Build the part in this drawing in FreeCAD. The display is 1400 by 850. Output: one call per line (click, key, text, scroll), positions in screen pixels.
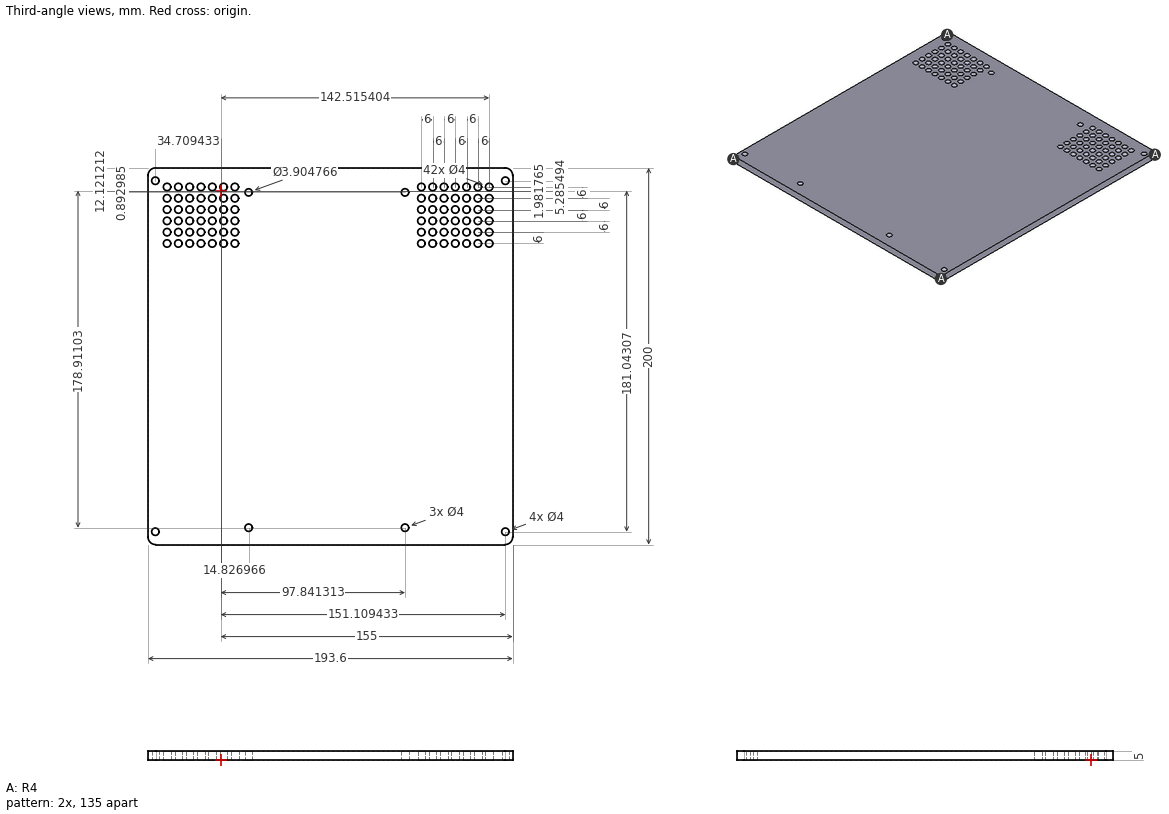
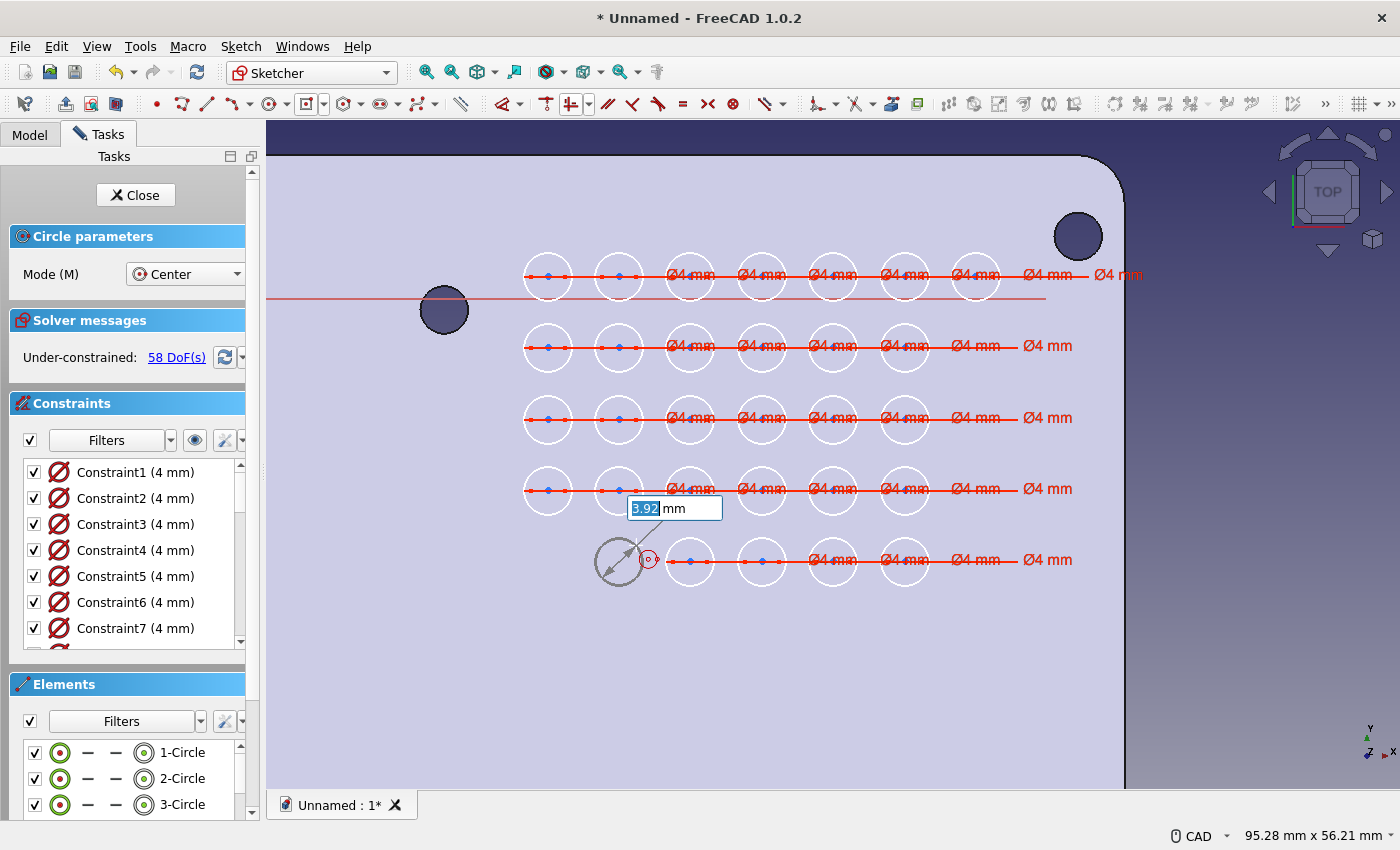
text(4)
key(Return)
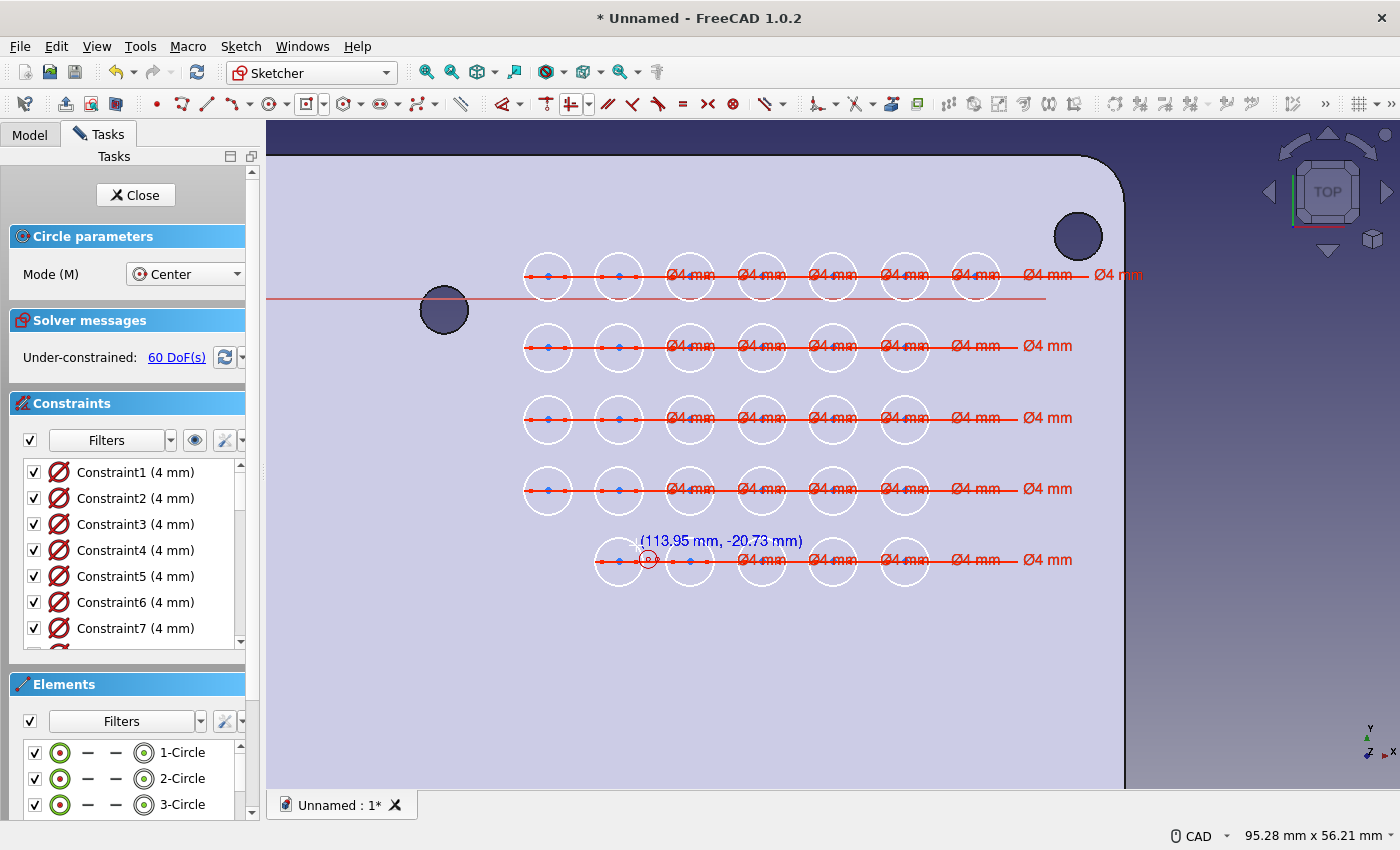
click(548, 561)
move(564, 545)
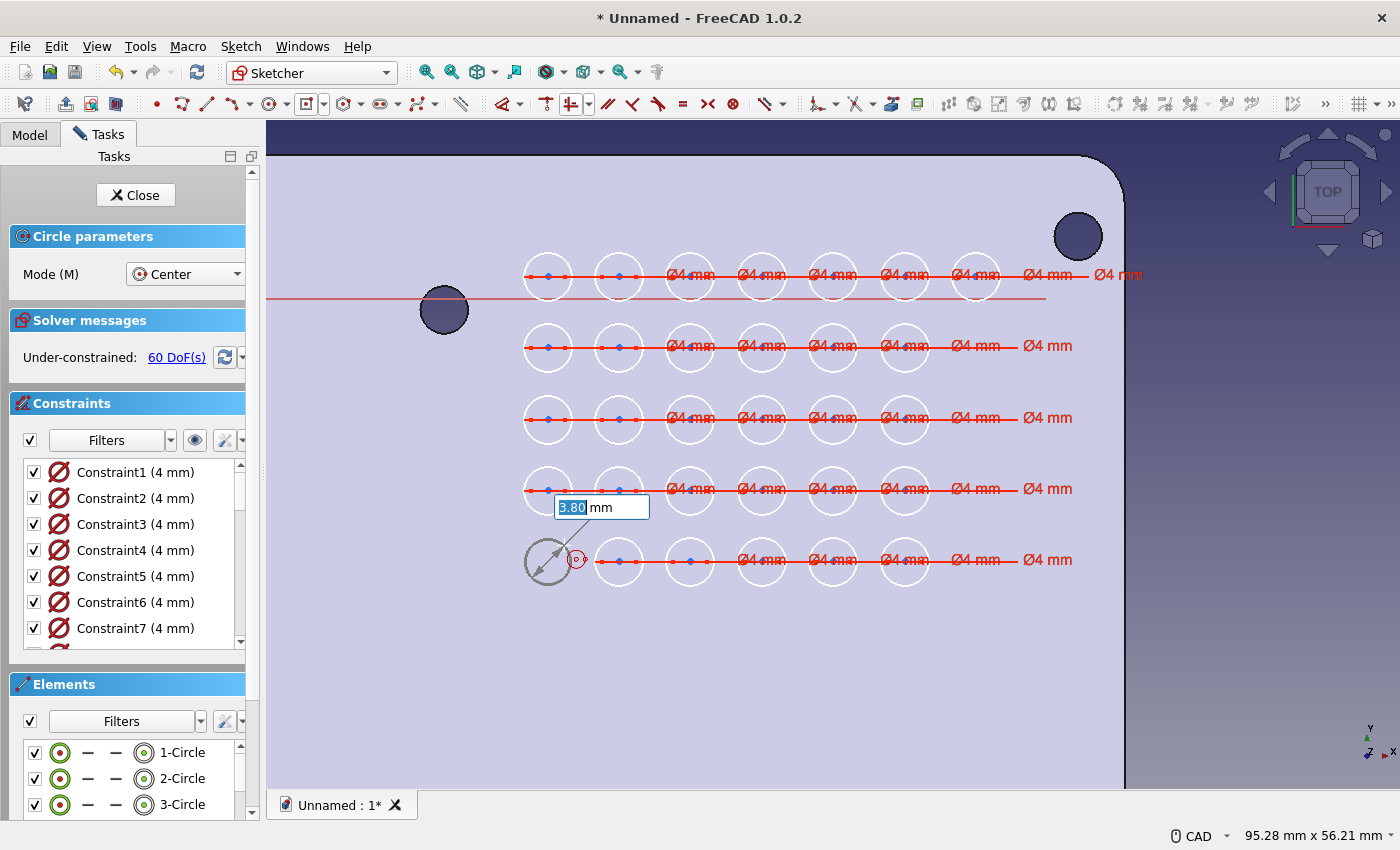
text(4)
key(Return)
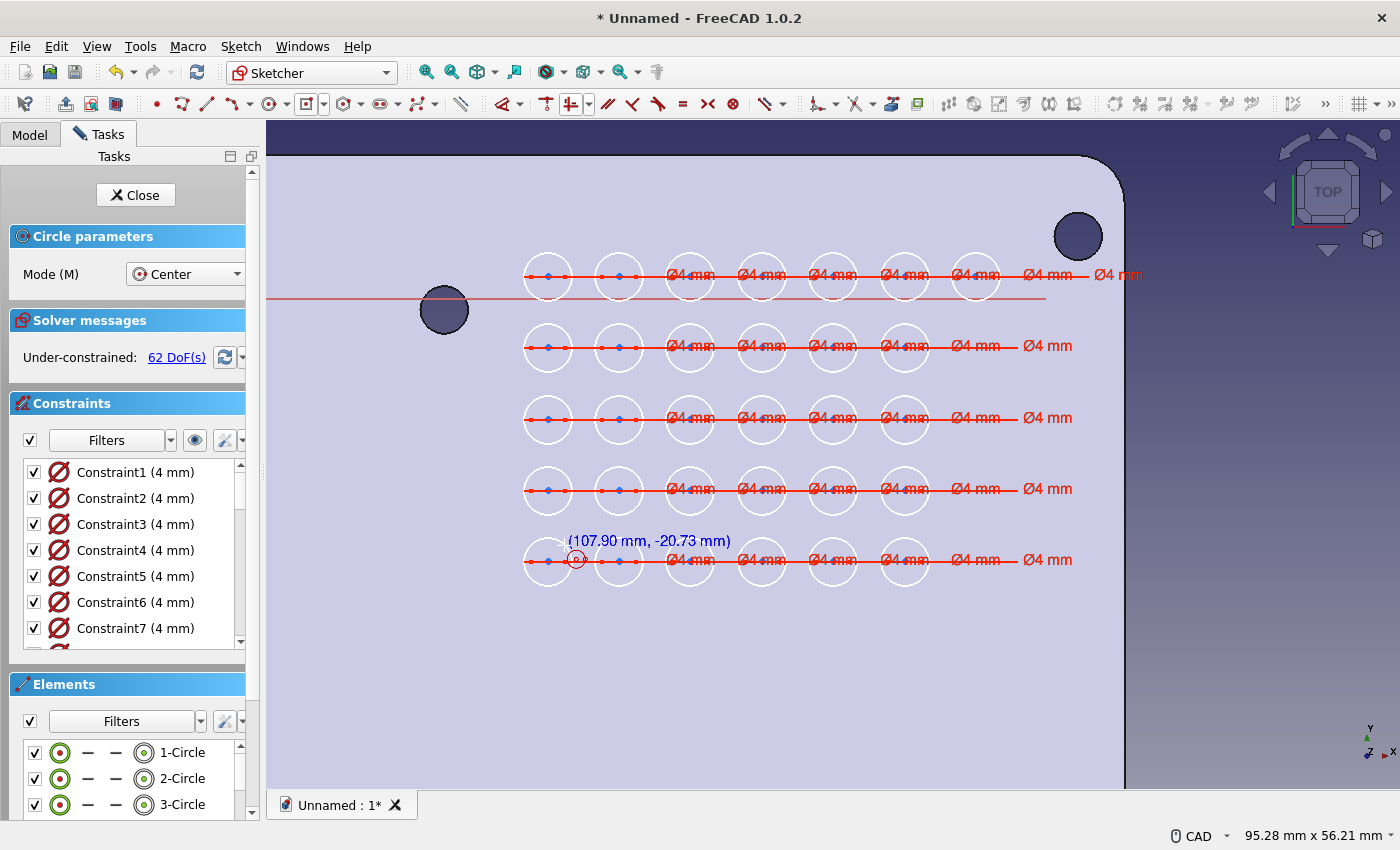
click(905, 633)
move(921, 616)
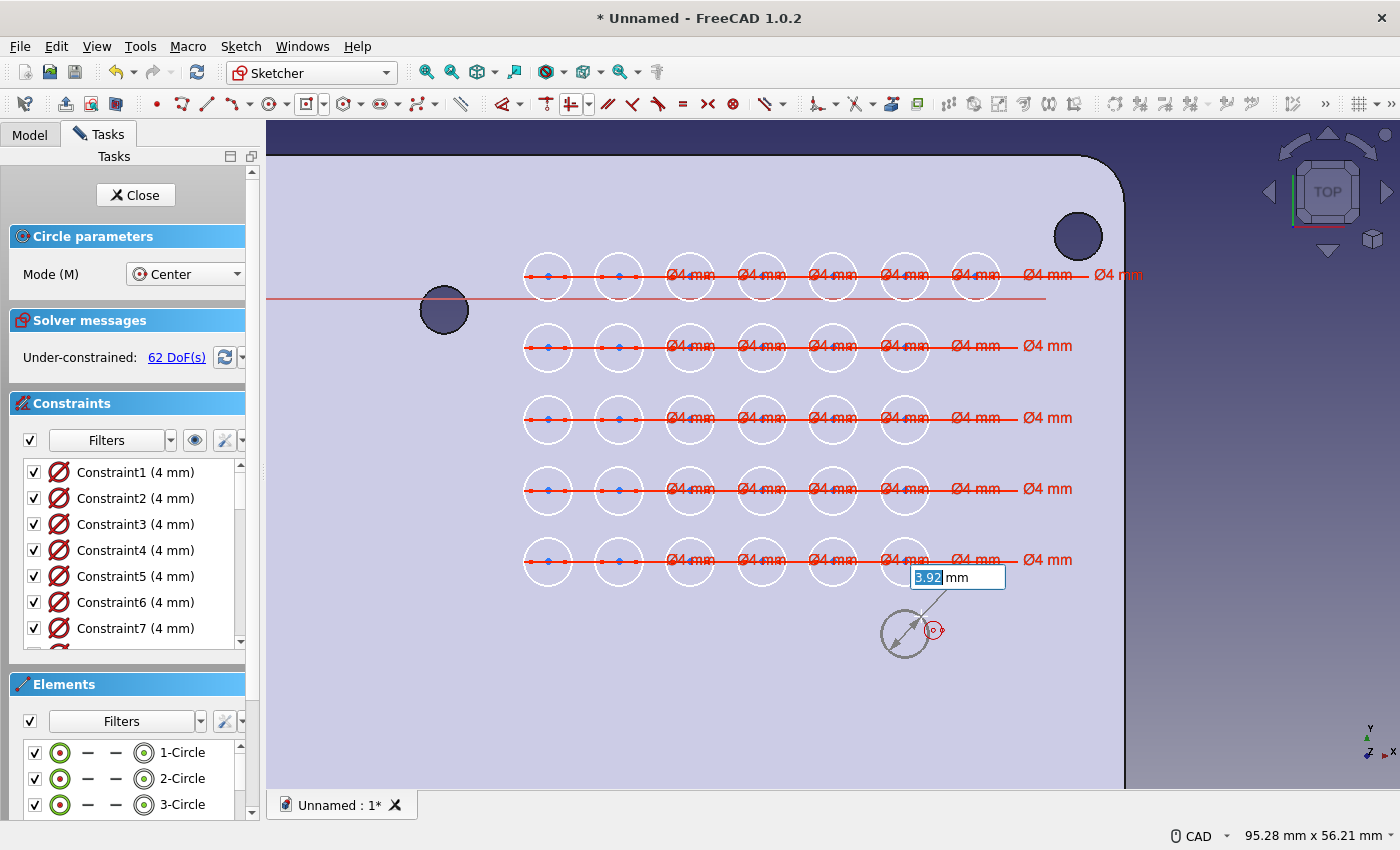
text(4)
key(Return)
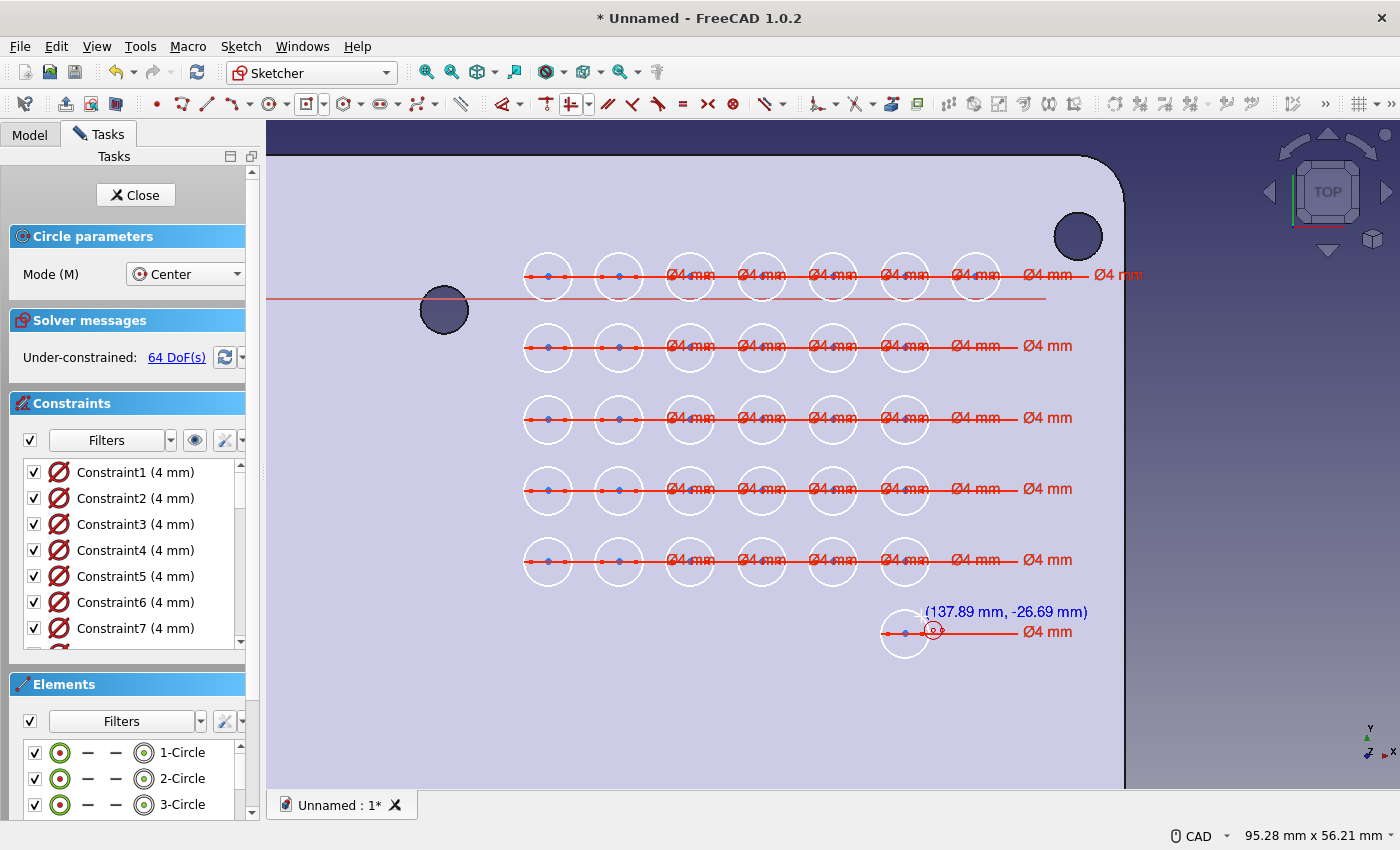
click(833, 633)
move(850, 616)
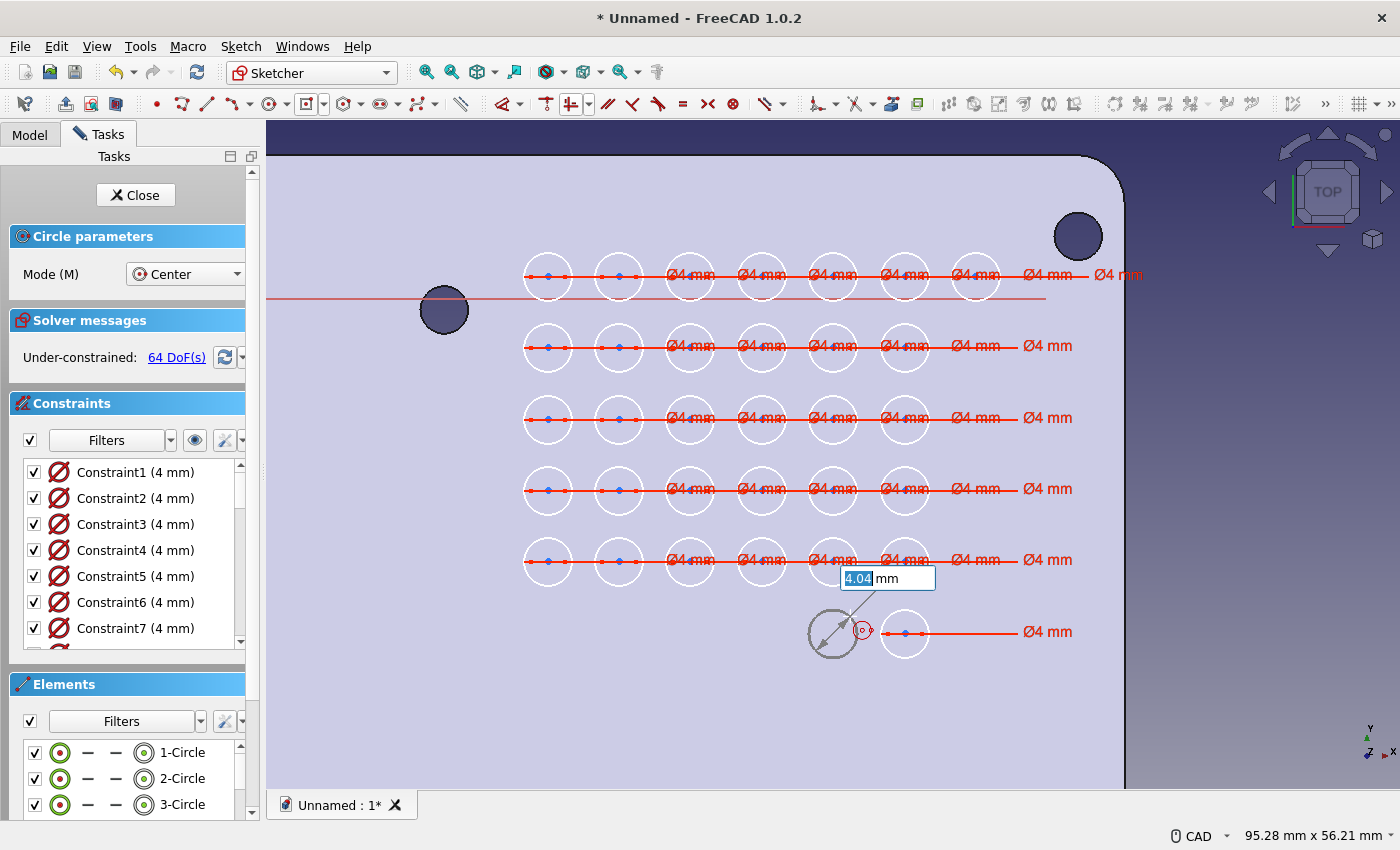
text(4)
key(Return)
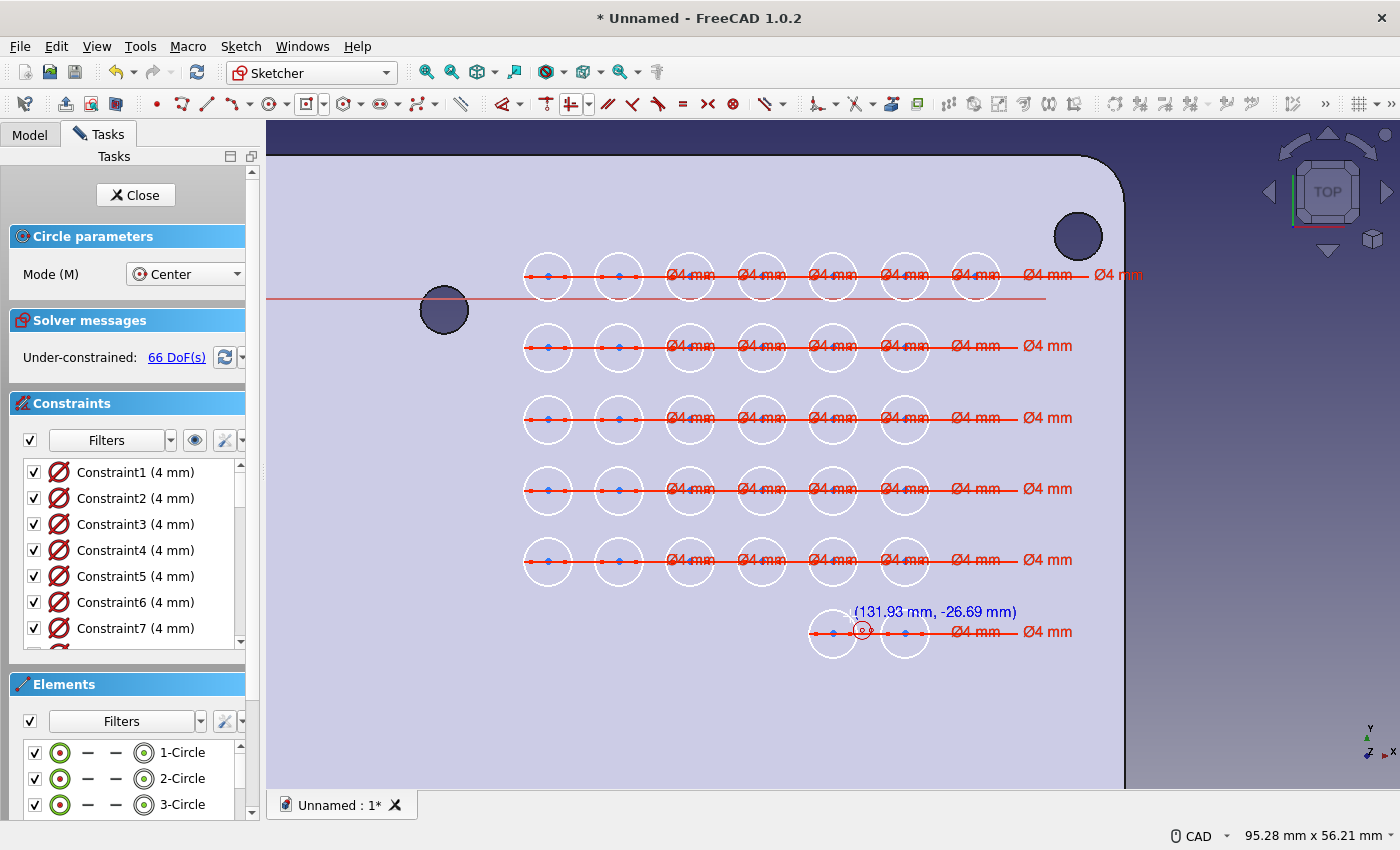
click(762, 633)
move(779, 616)